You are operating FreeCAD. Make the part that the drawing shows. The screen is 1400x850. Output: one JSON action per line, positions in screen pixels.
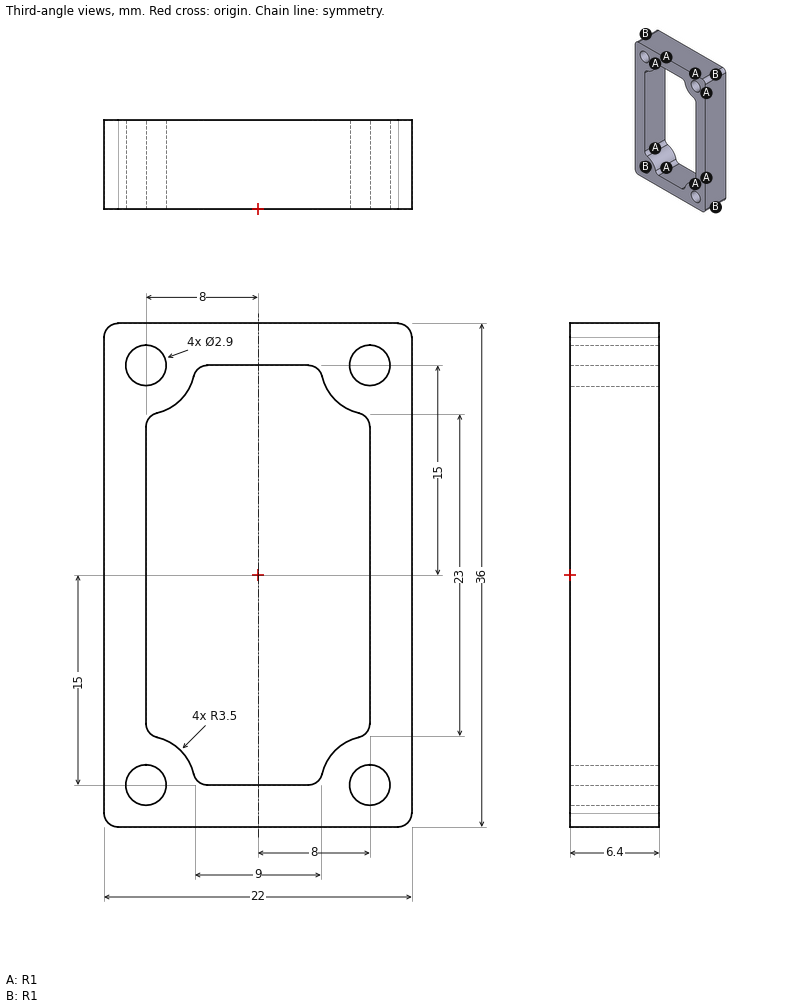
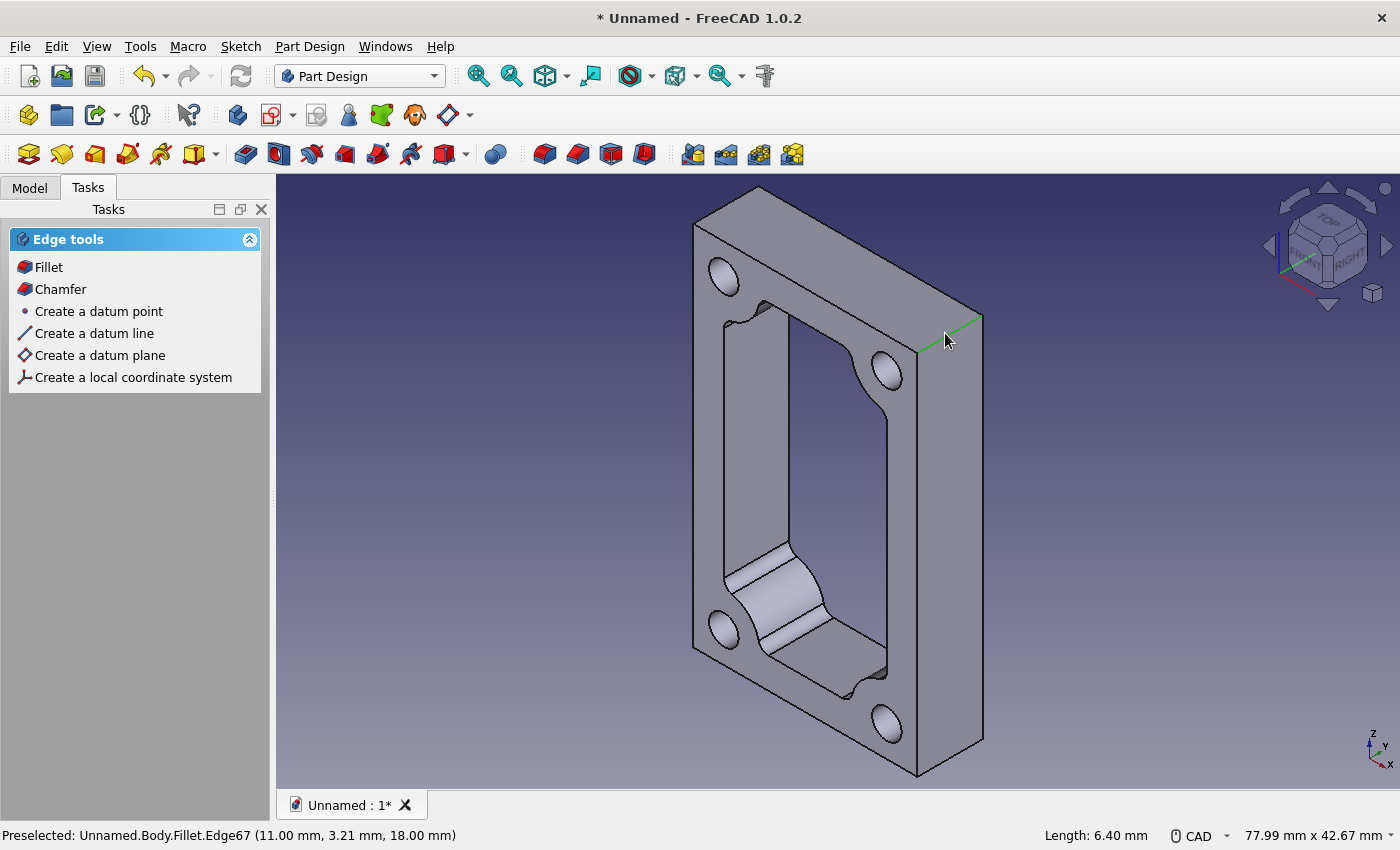
{"action": "key", "text": "2"}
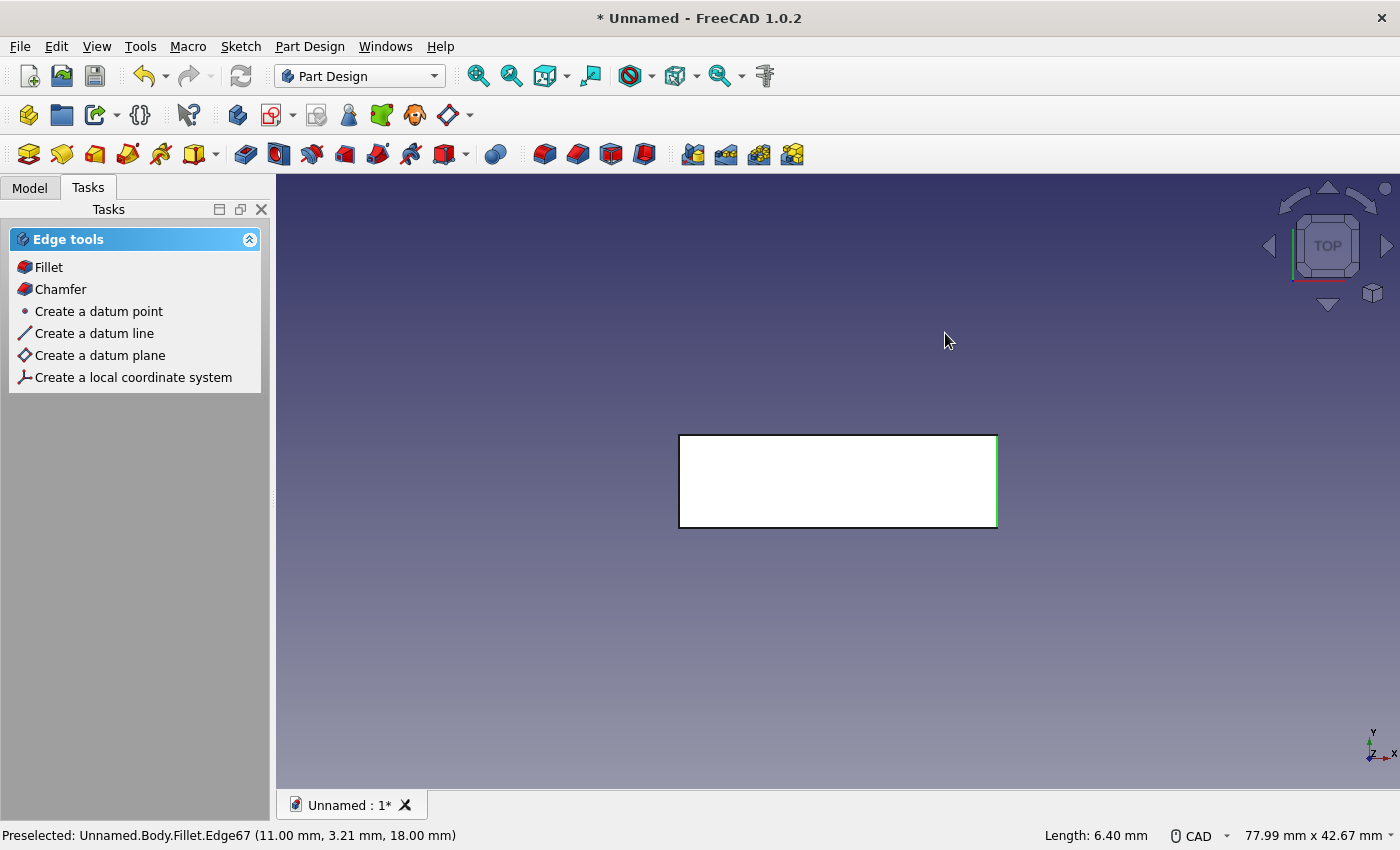
{"action": "left_click", "coordinate": [479, 76]}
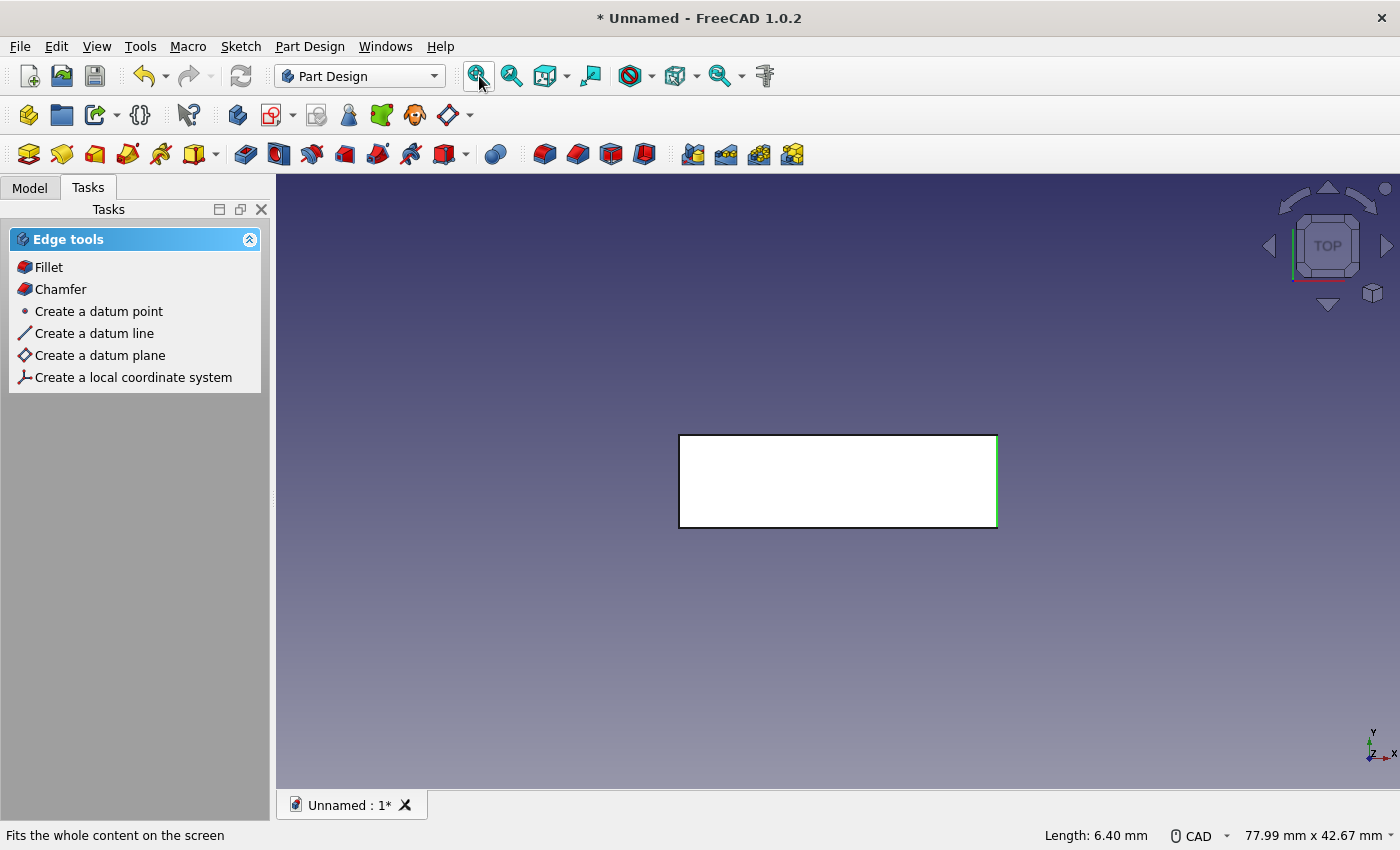
{"action": "left_click", "coordinate": [679, 481], "text": "ctrl"}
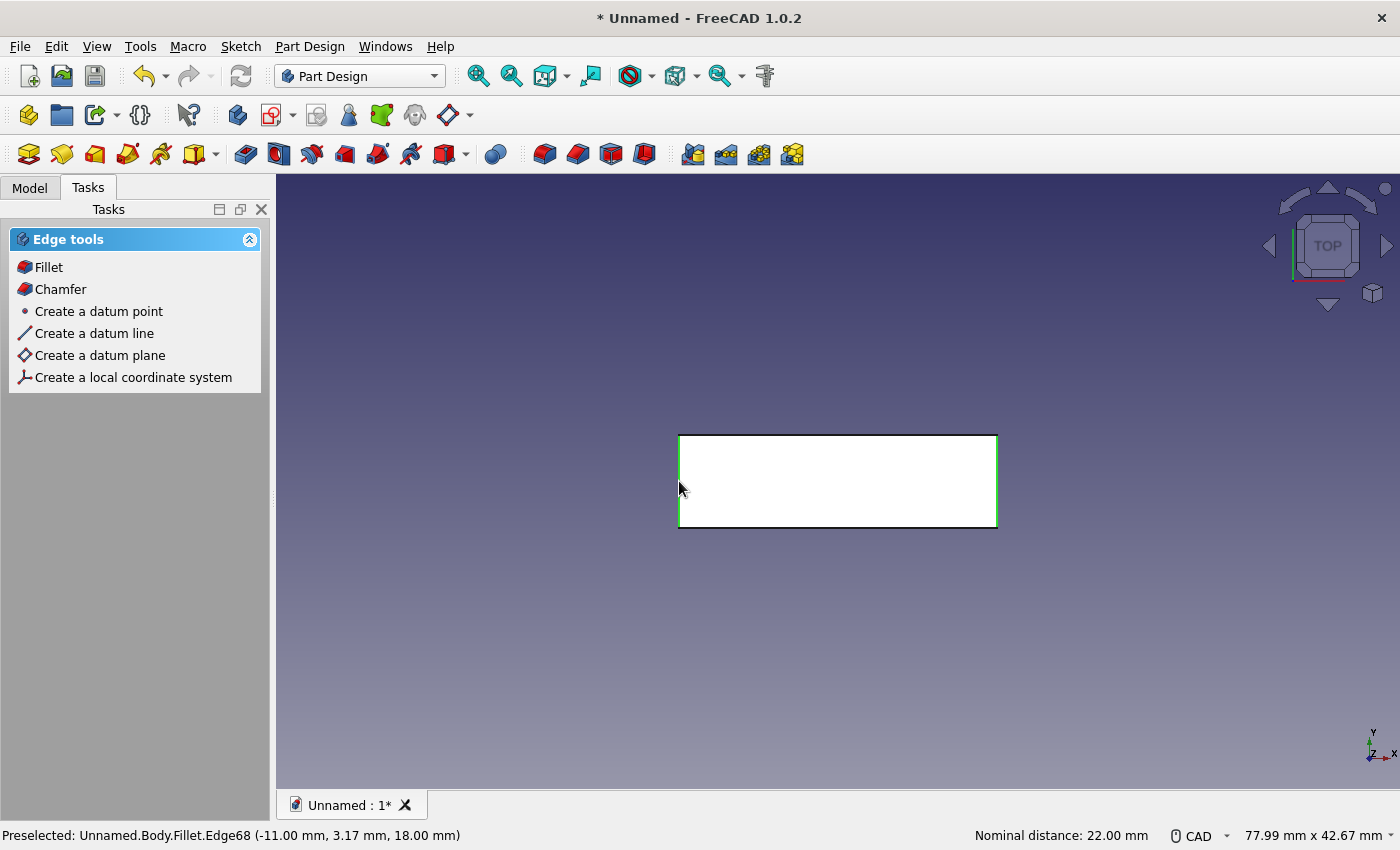
{"action": "key", "text": "0"}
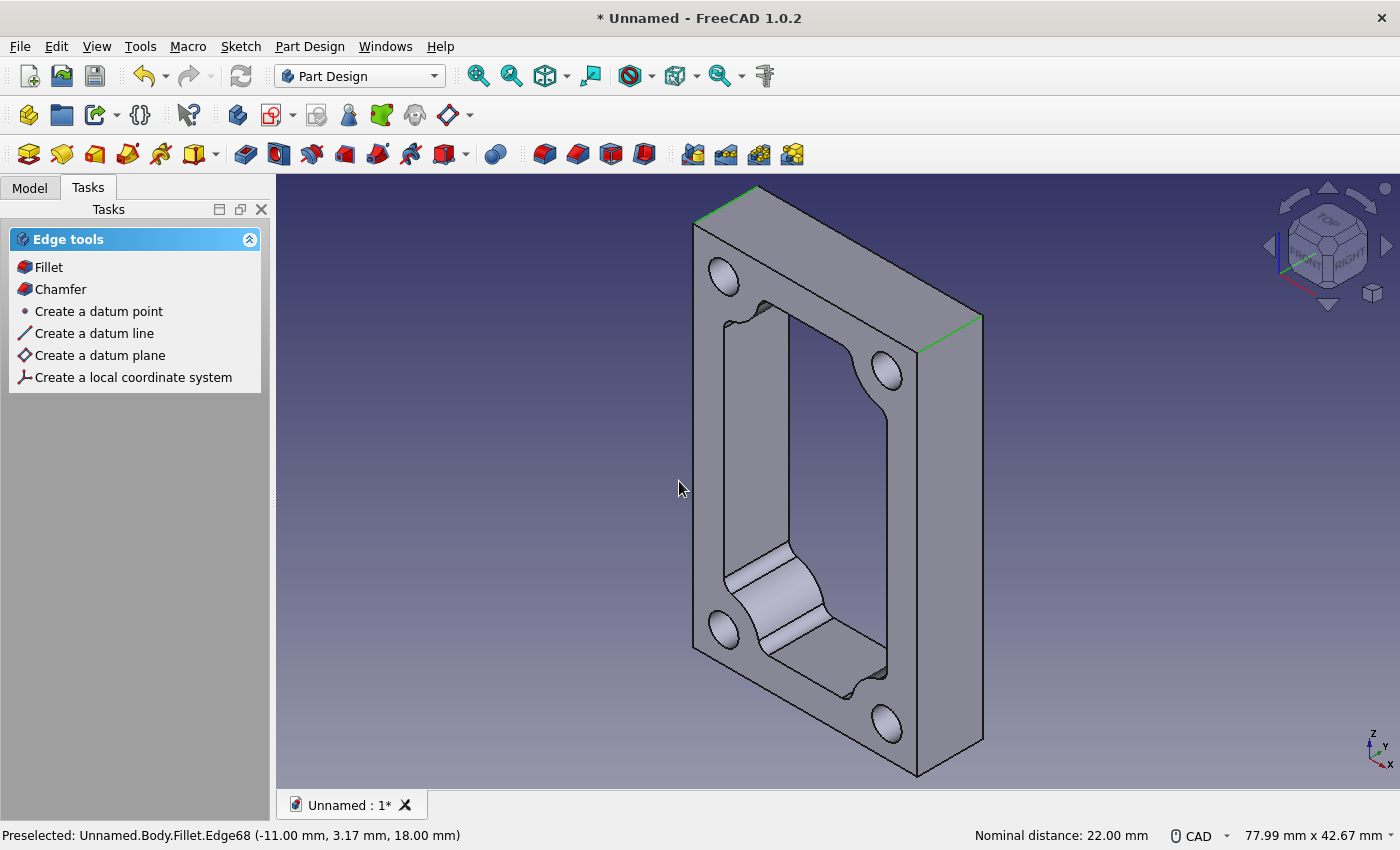
{"action": "key", "text": "1"}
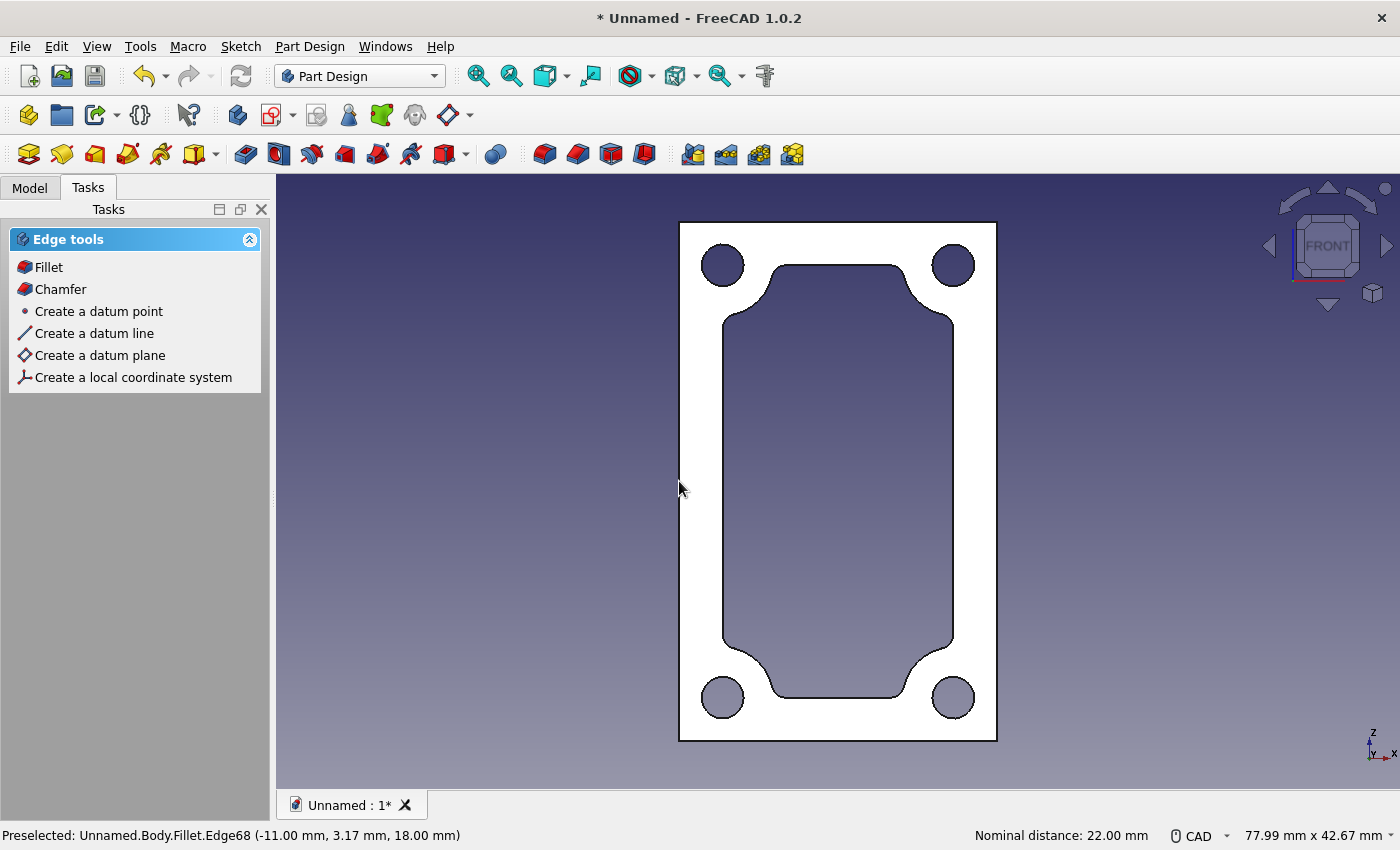
{"action": "key", "text": "3"}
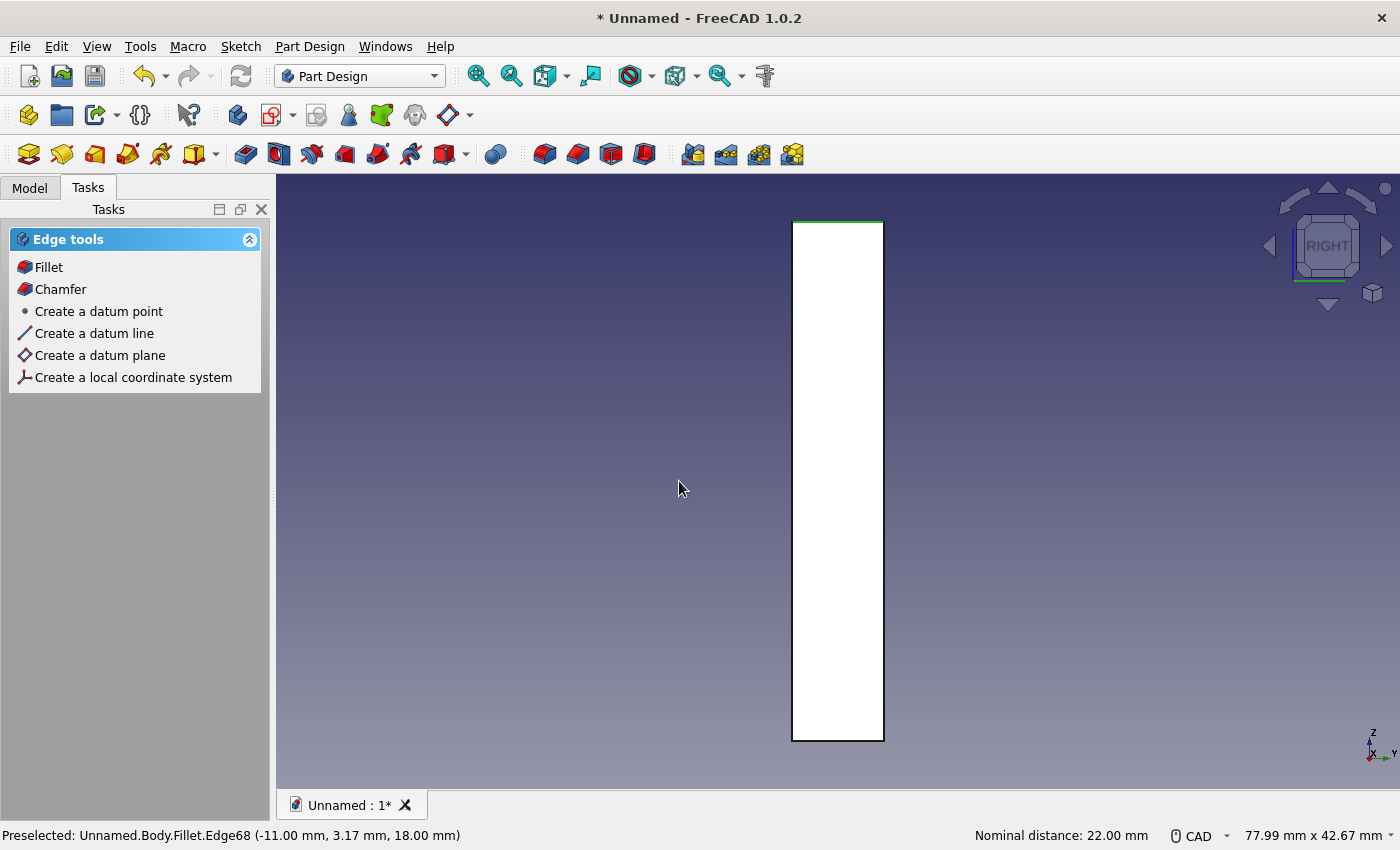
{"action": "left_click", "coordinate": [838, 740], "text": "ctrl"}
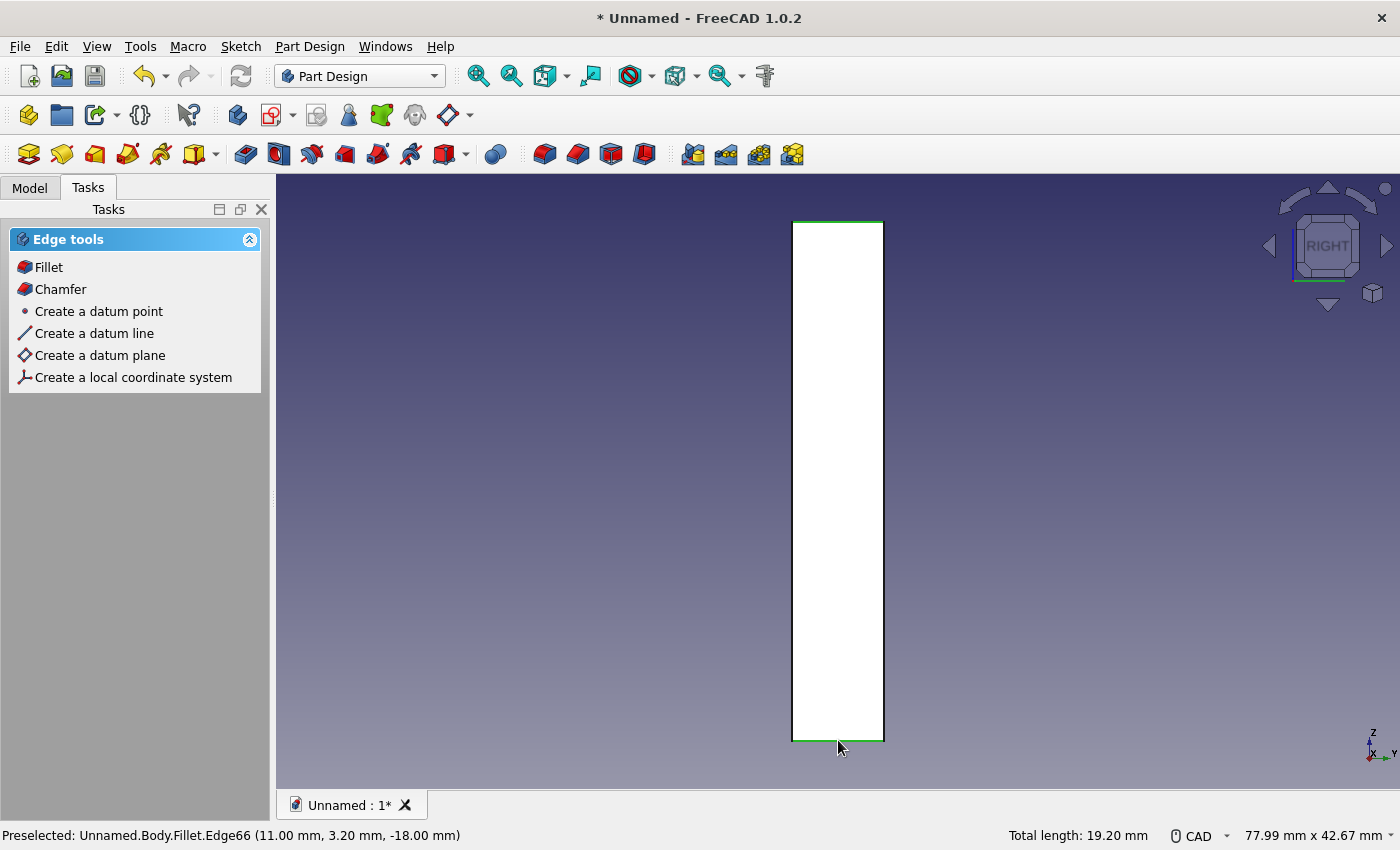
{"action": "key", "text": "5"}